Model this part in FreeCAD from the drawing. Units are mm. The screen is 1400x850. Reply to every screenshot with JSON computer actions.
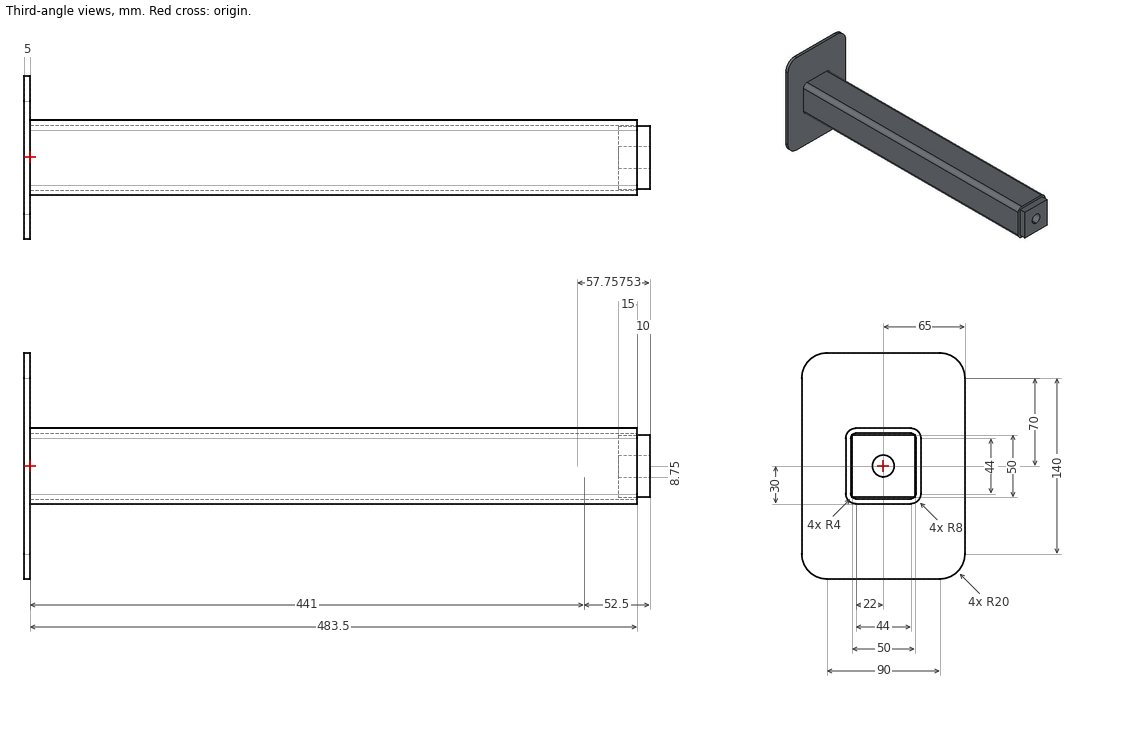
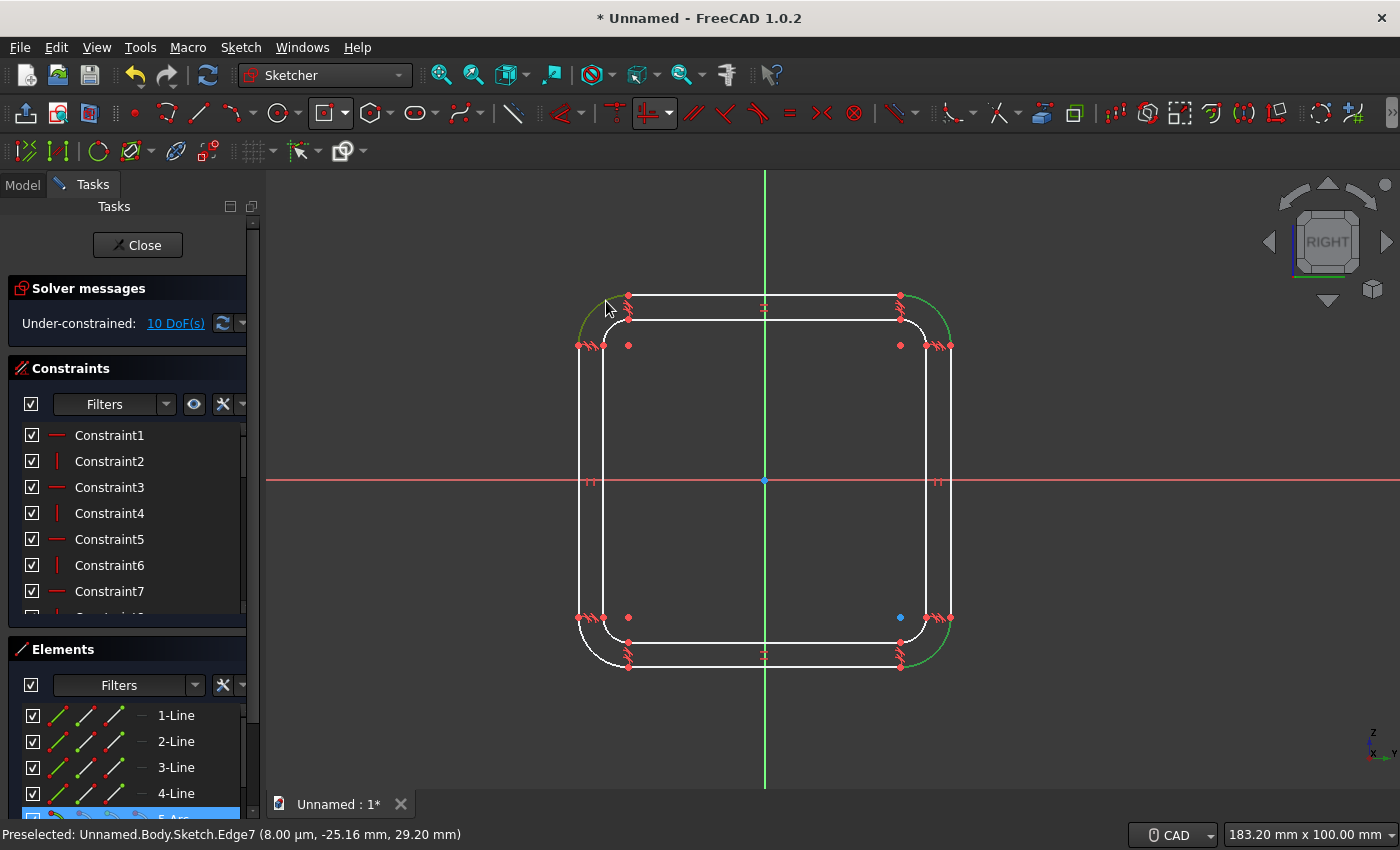
{"action": "left_click", "coordinate": [584, 640]}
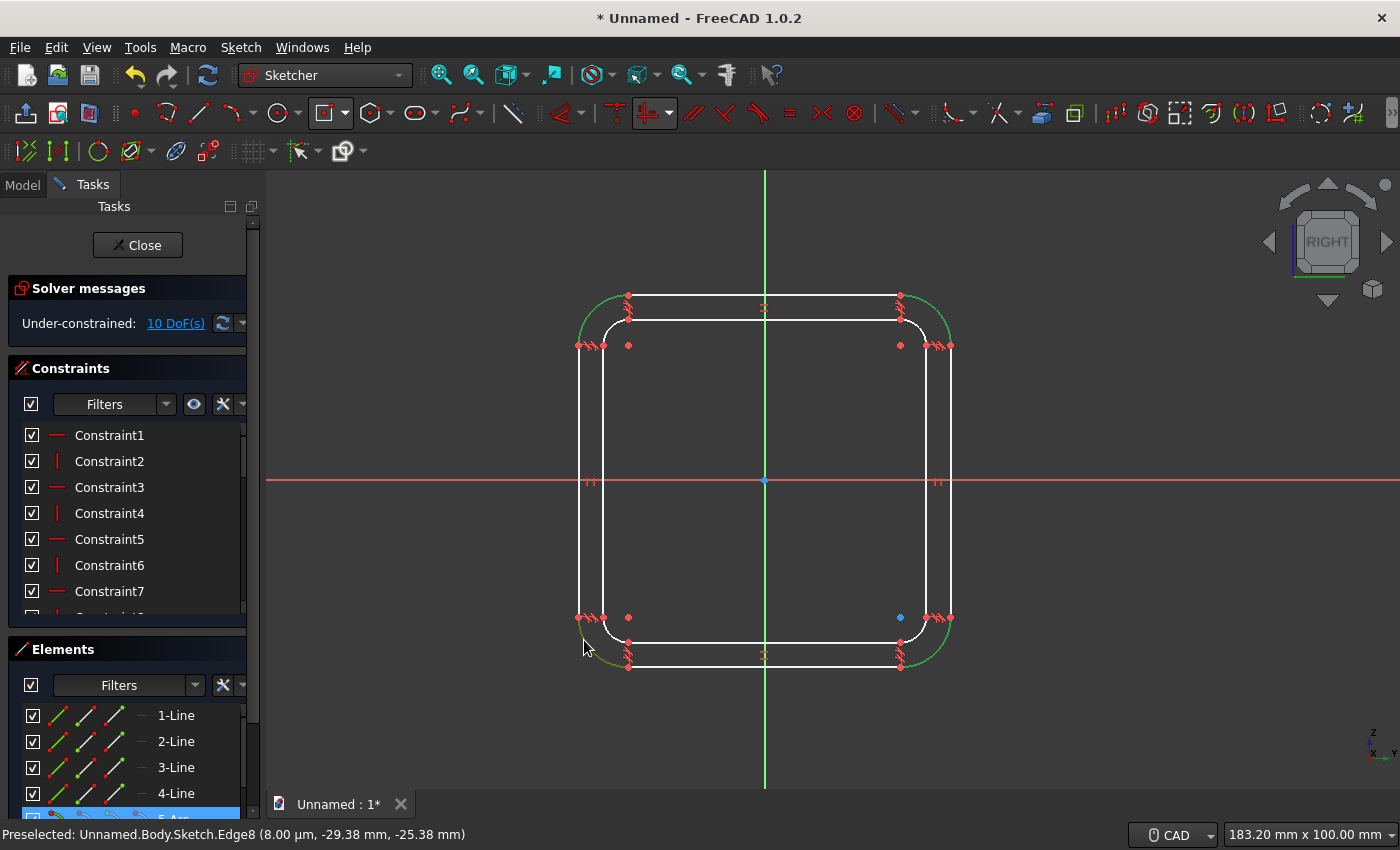
{"action": "left_click", "coordinate": [790, 114]}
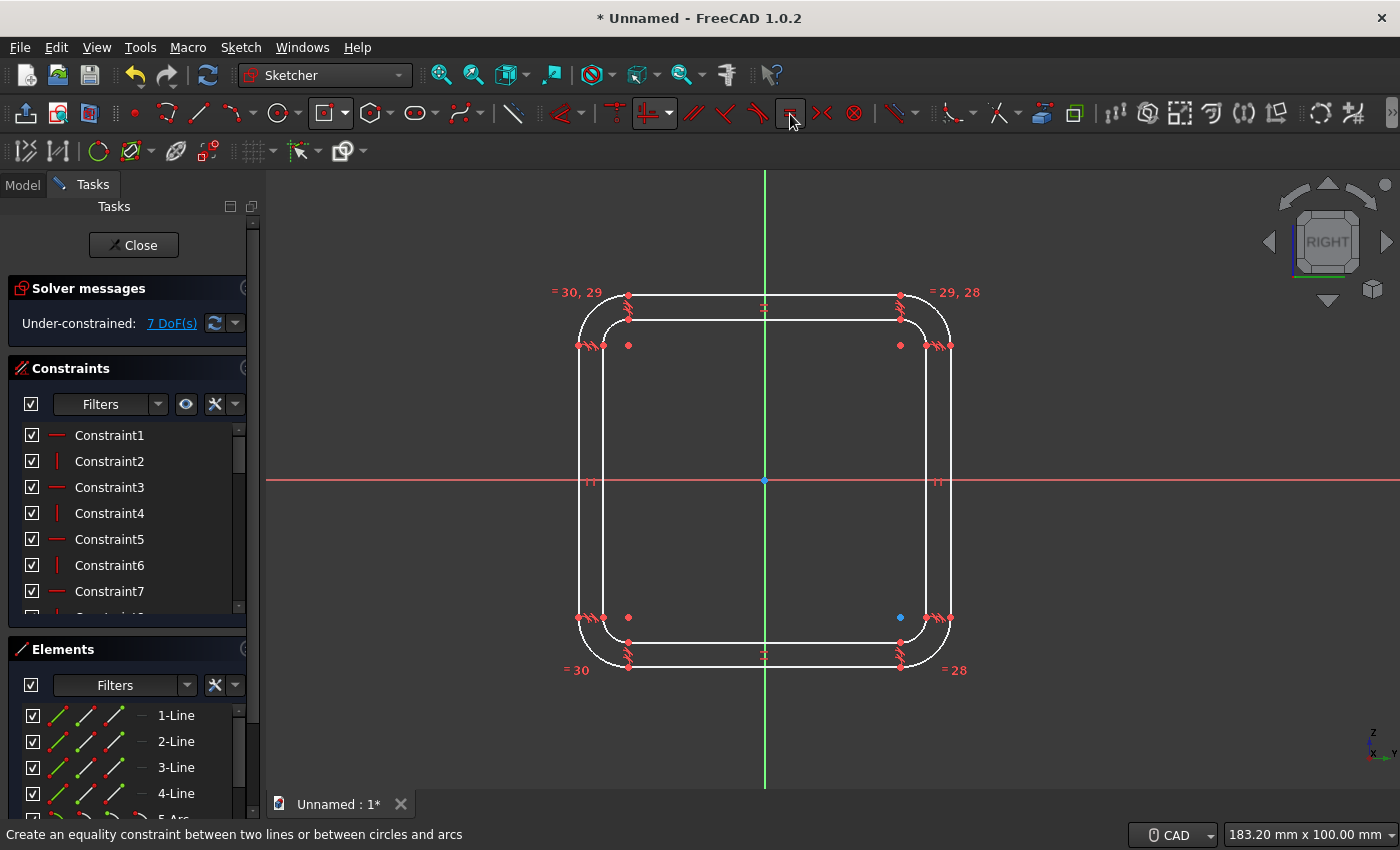
{"action": "left_click", "coordinate": [606, 629]}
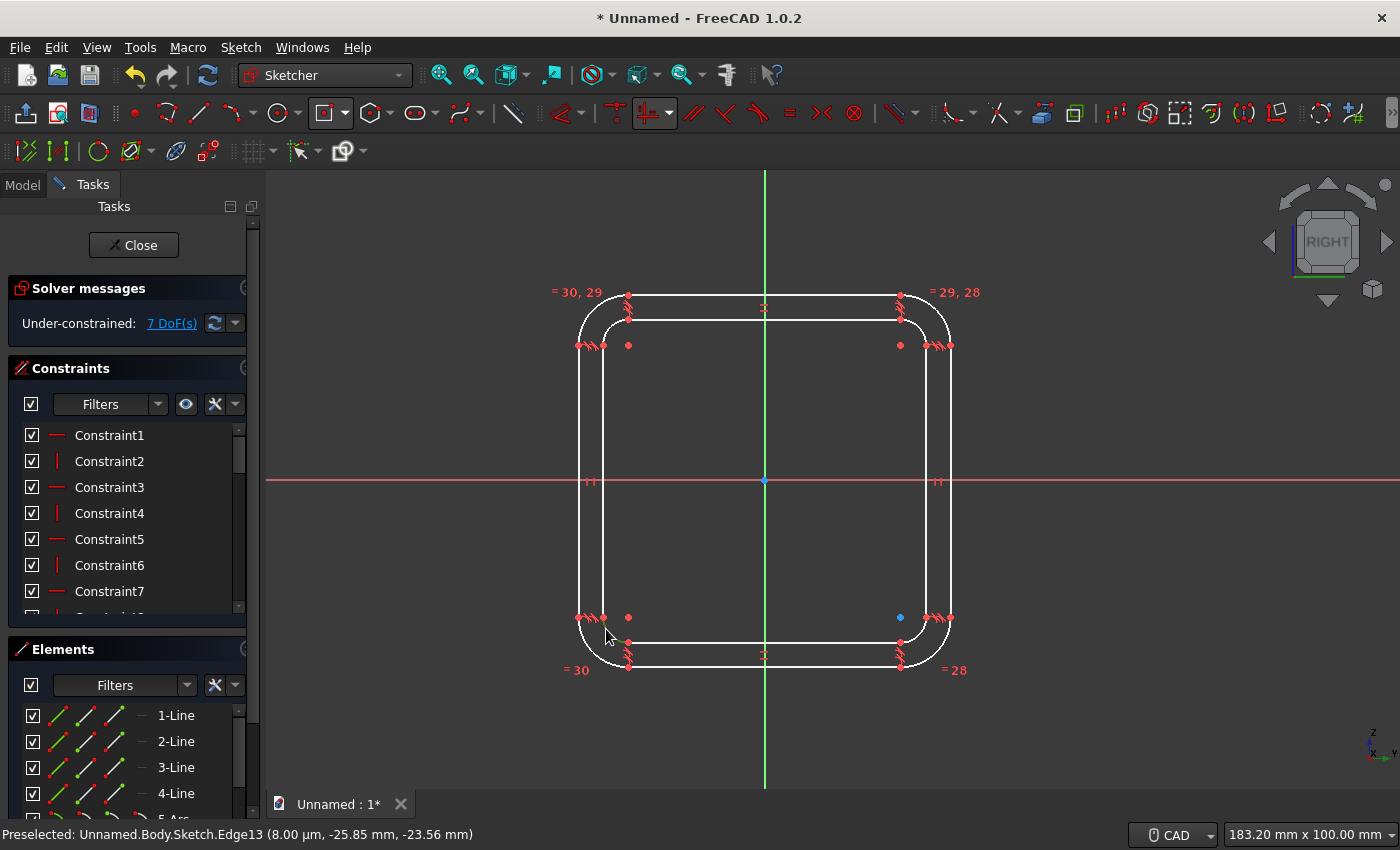
{"action": "left_click", "coordinate": [912, 640]}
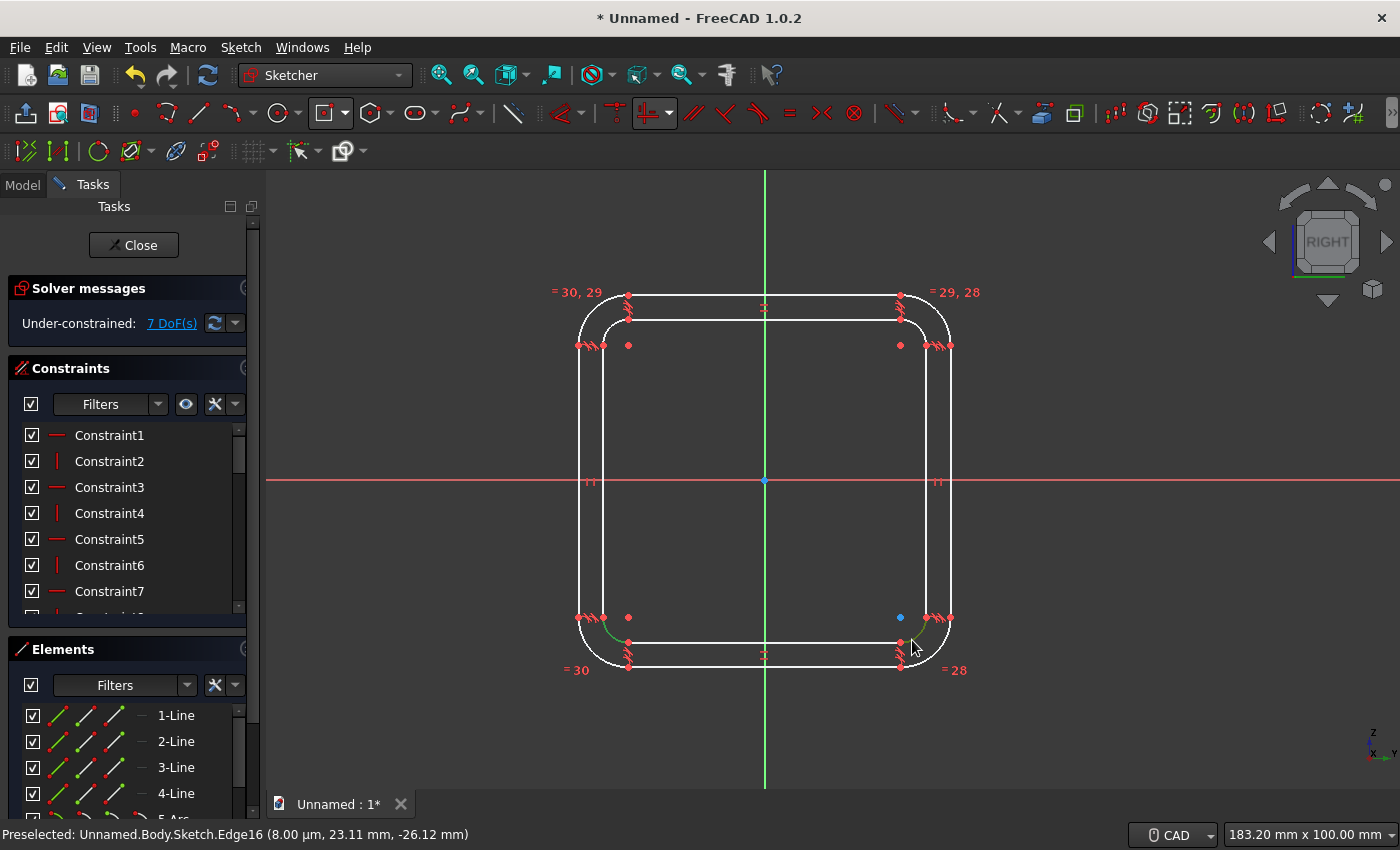
{"action": "left_click", "coordinate": [790, 114]}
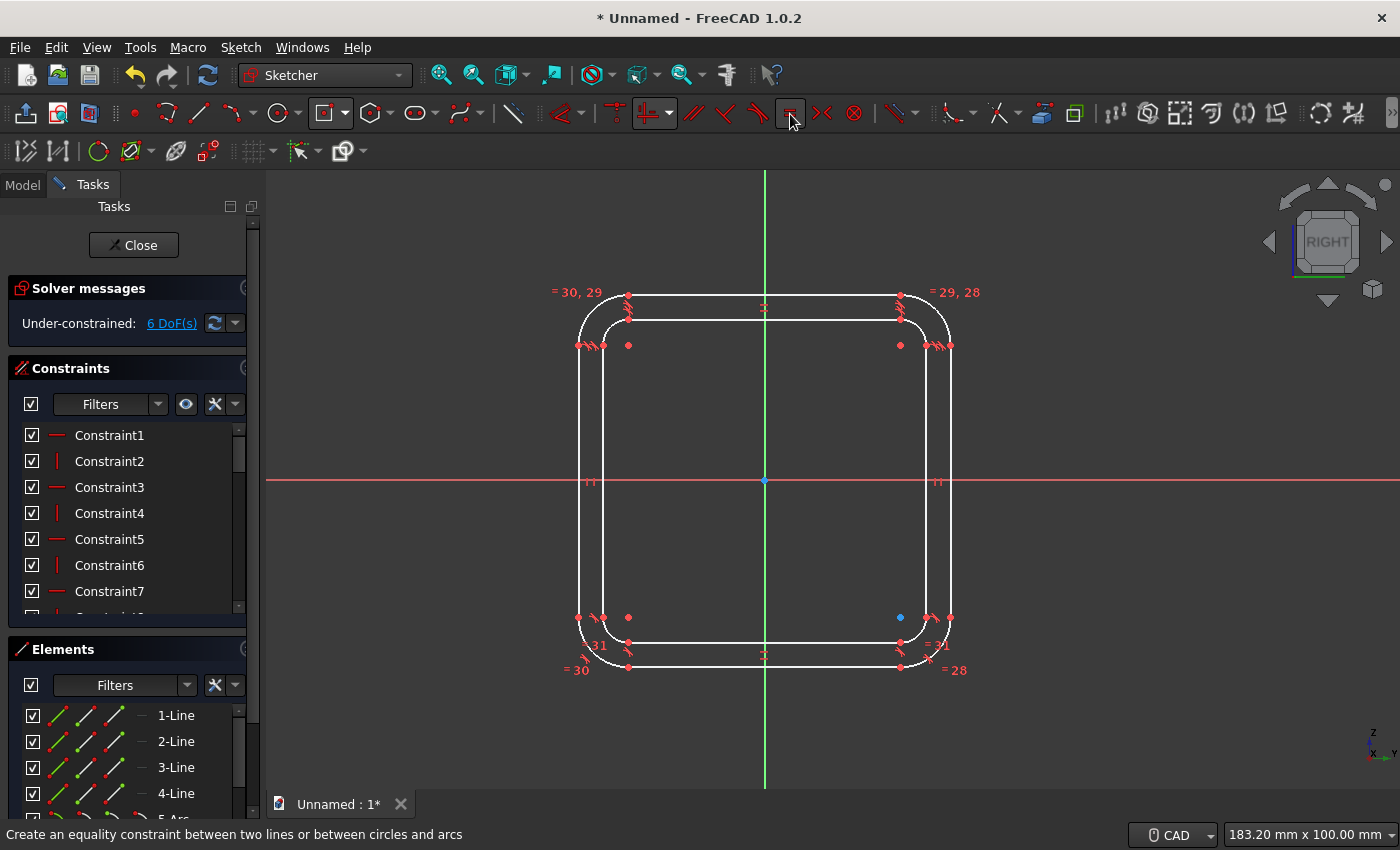
{"action": "left_click", "coordinate": [916, 665]}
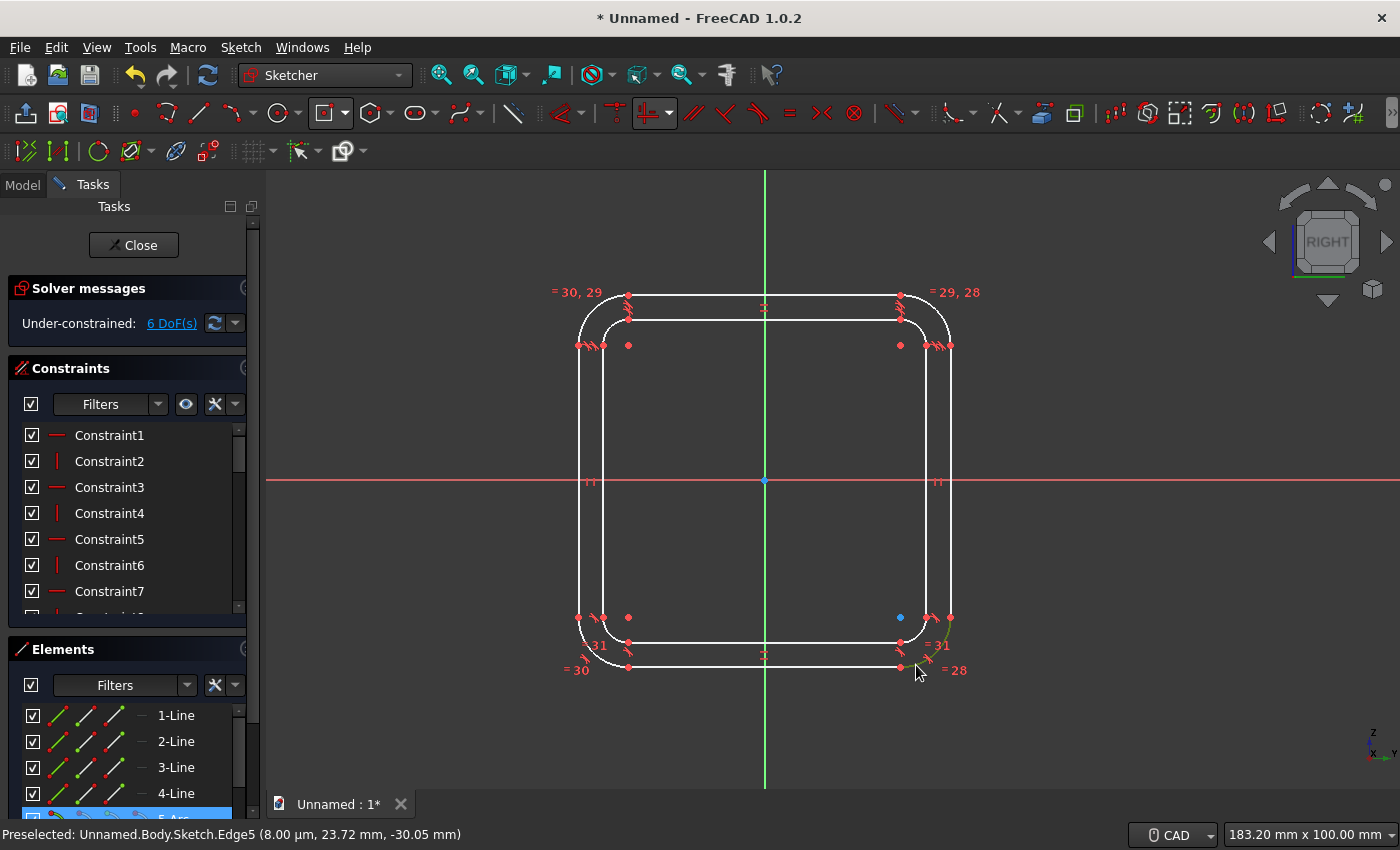
{"action": "key", "text": "k r"}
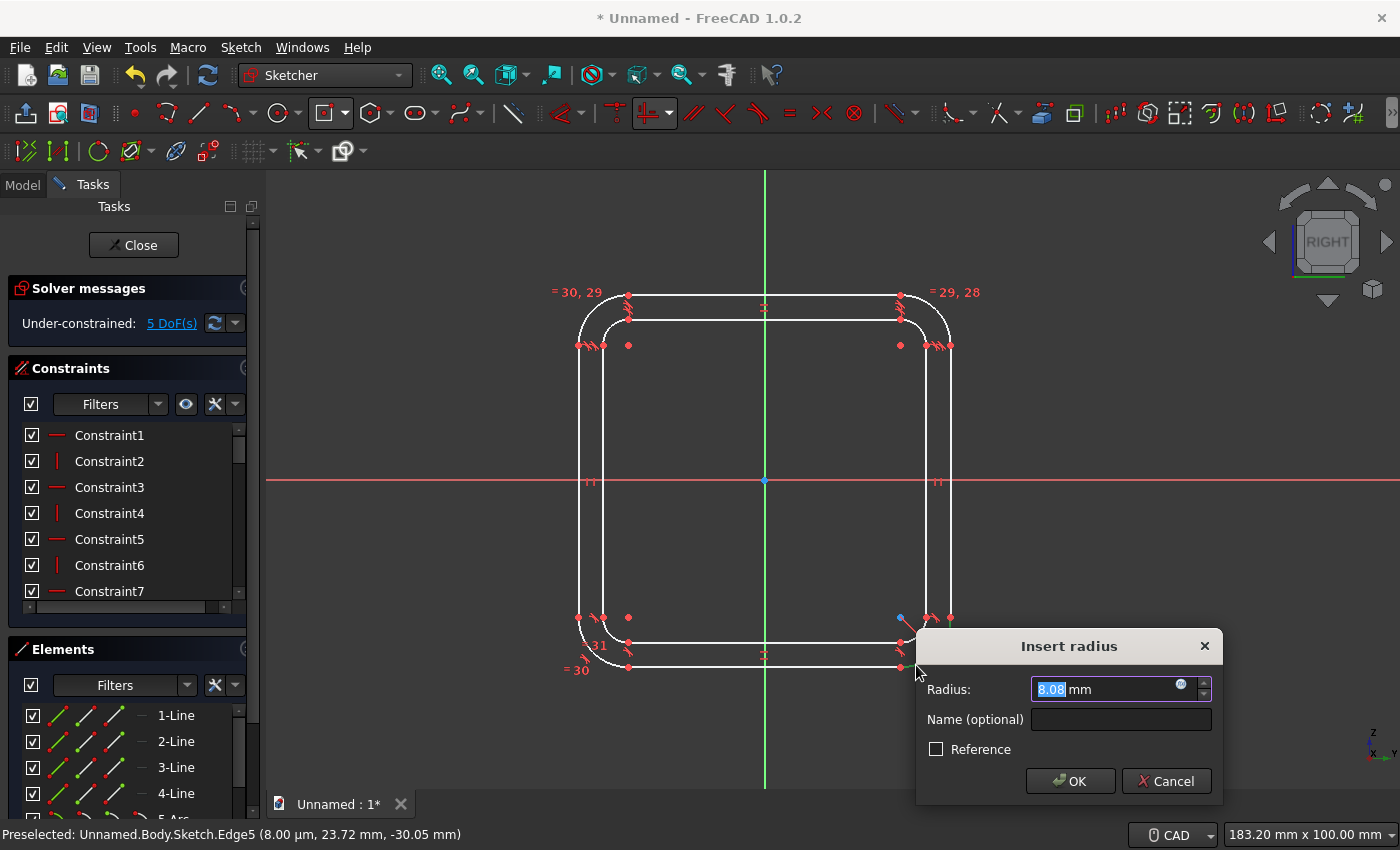
{"action": "type", "text": "8"}
{"action": "key", "text": "Return"}